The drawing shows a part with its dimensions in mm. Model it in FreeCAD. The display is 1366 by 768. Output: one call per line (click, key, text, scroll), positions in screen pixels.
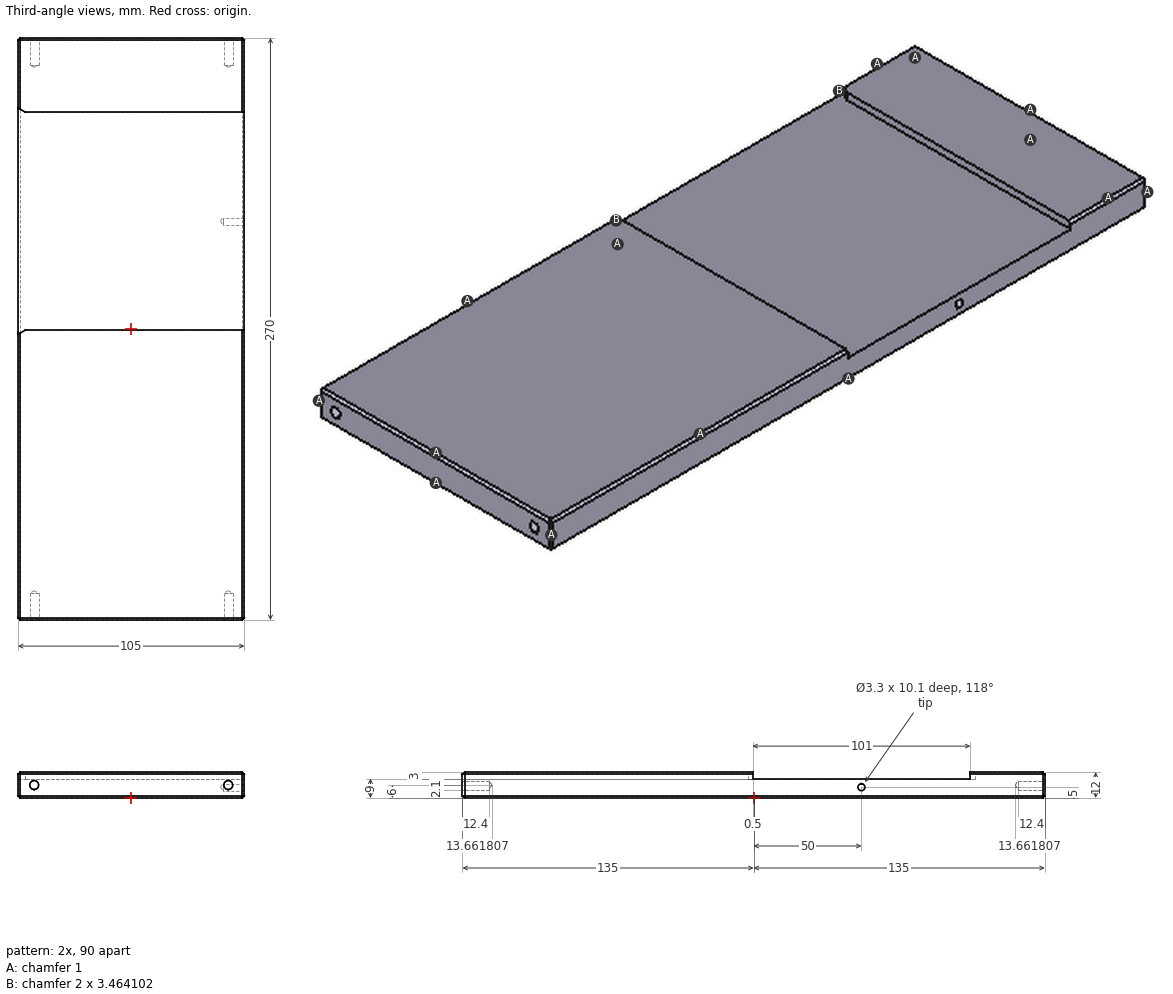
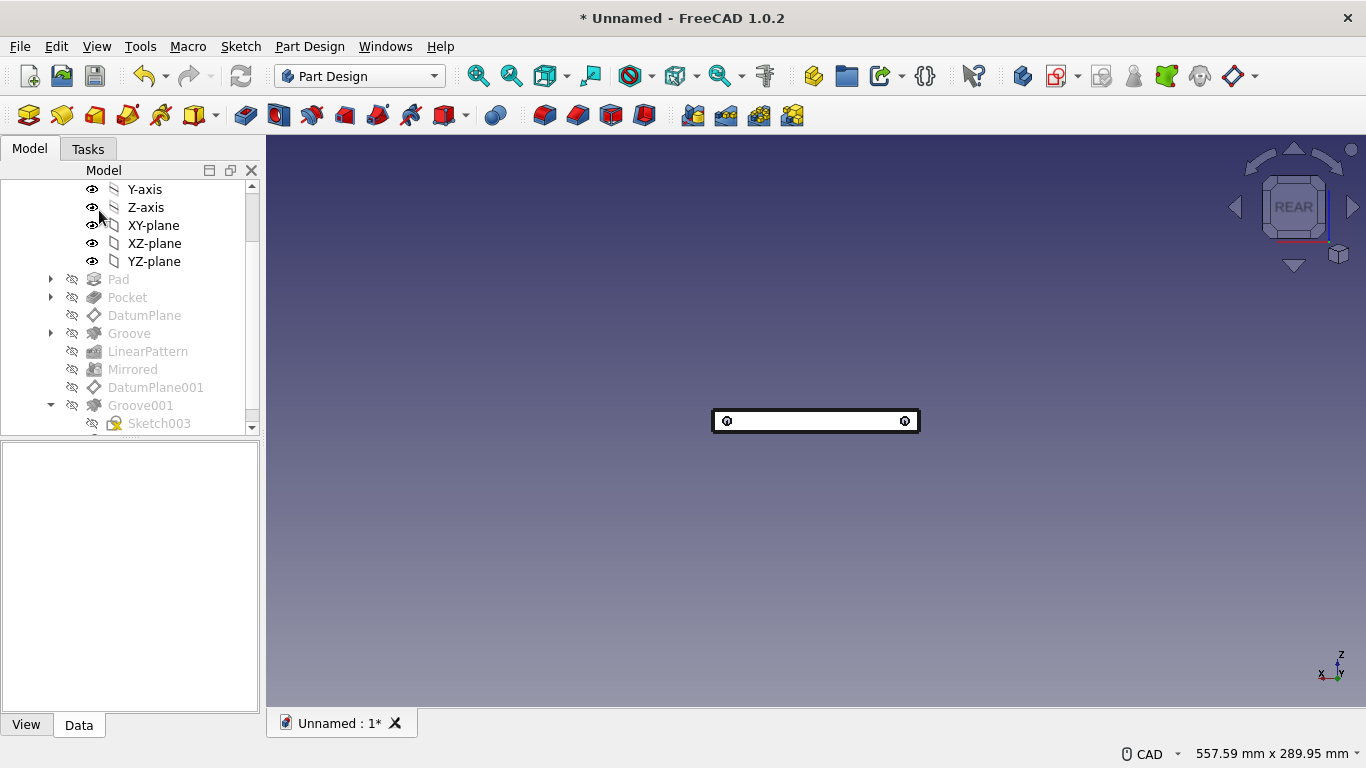
click(479, 76)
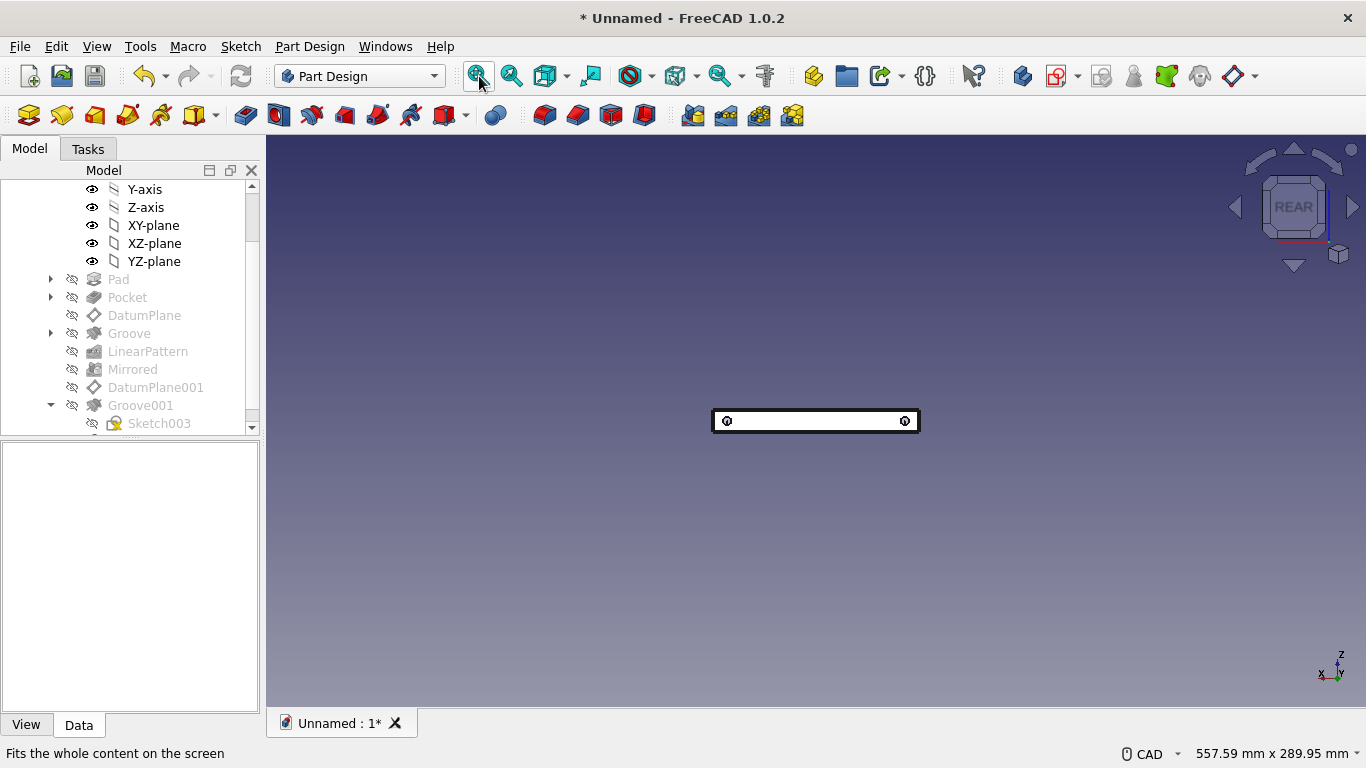
scroll(920, 412, up, 12)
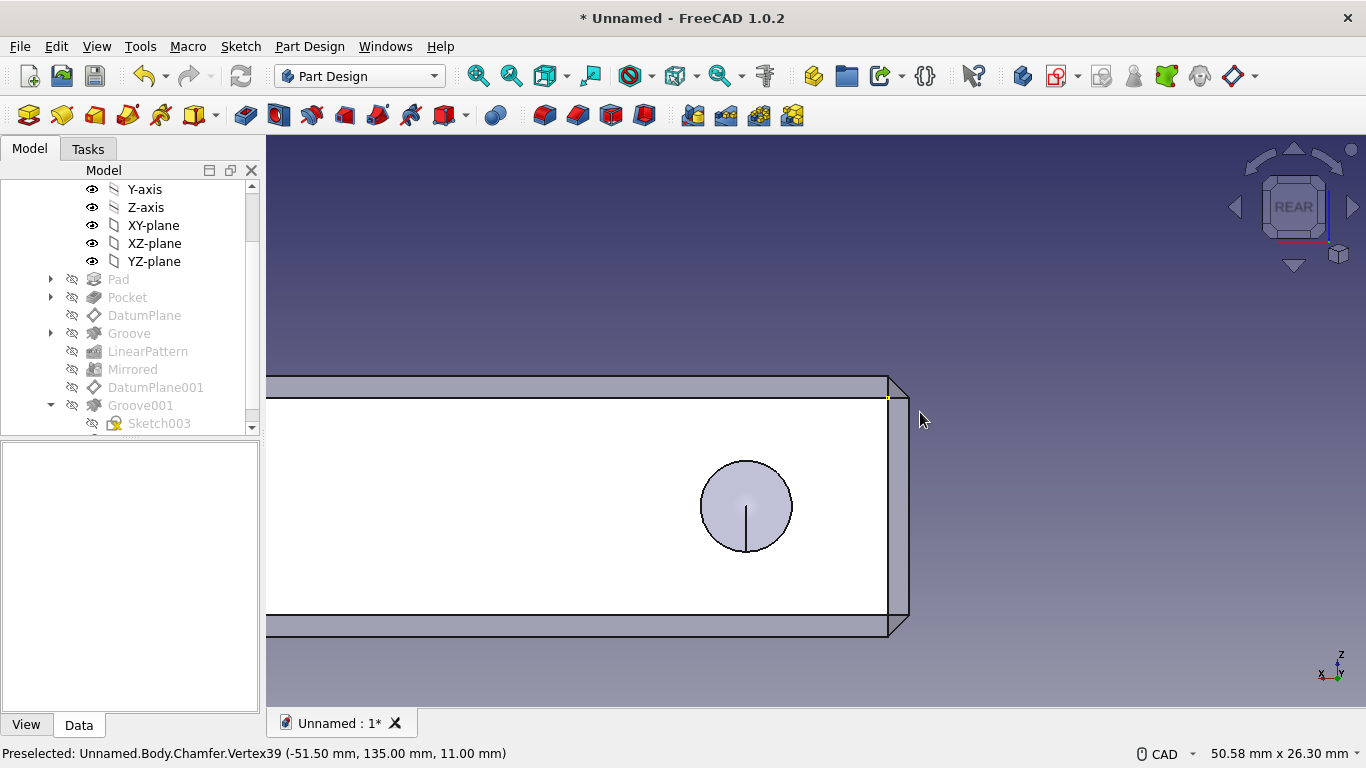
click(479, 76)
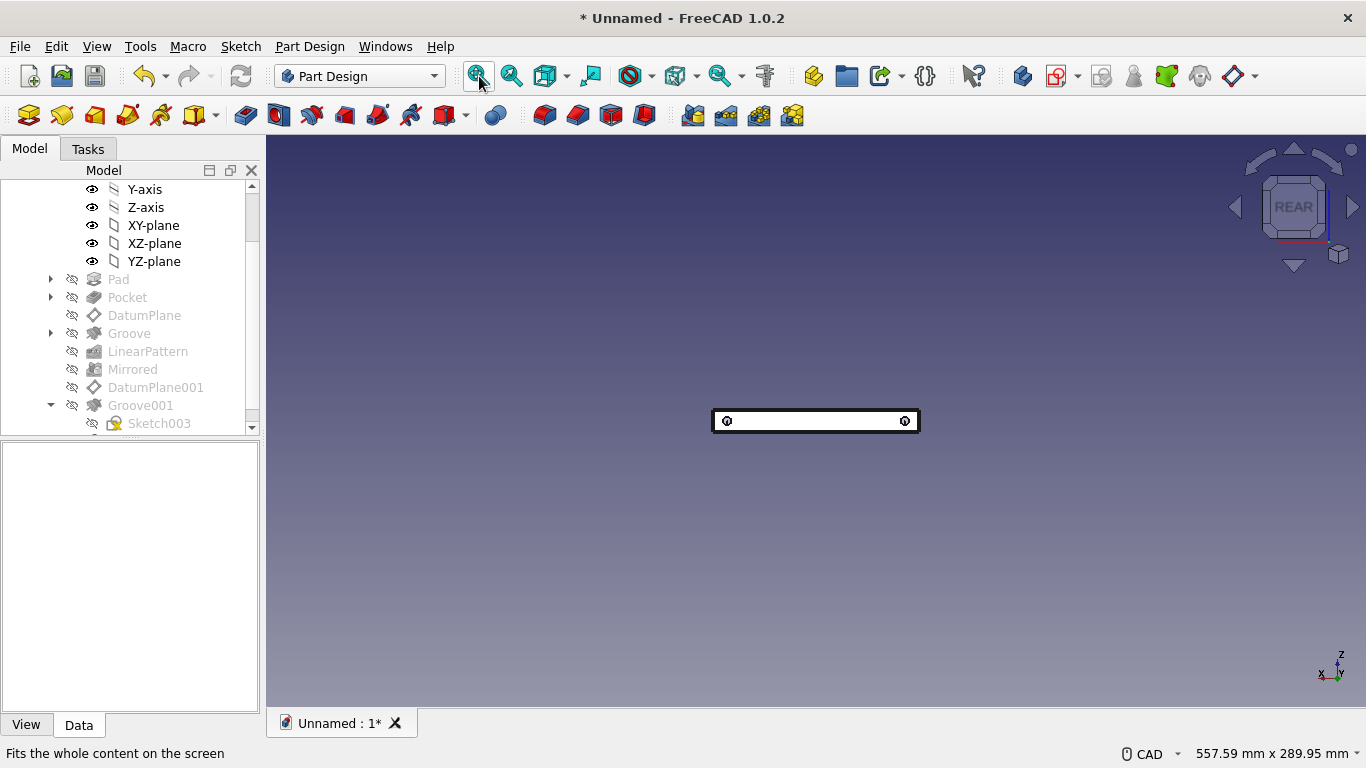
key(0)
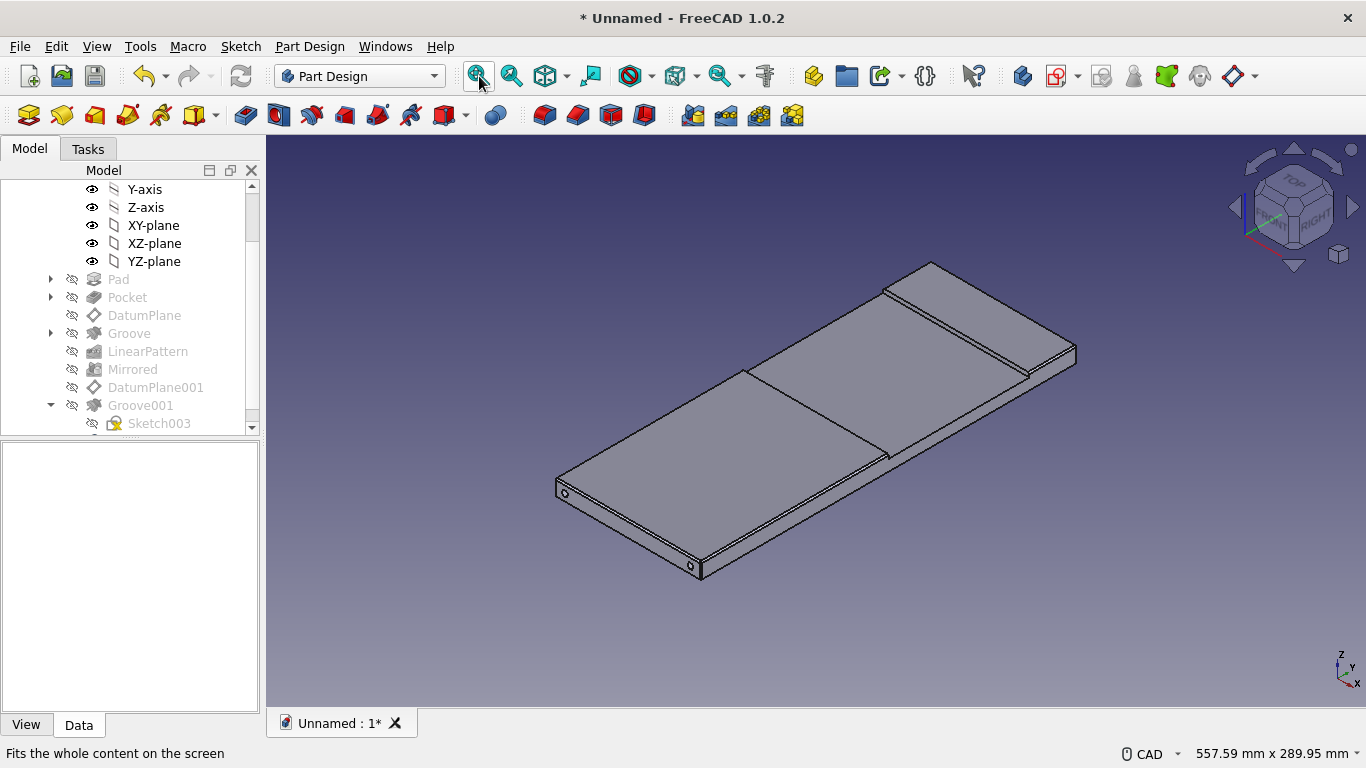
scroll(742, 372, up, 12)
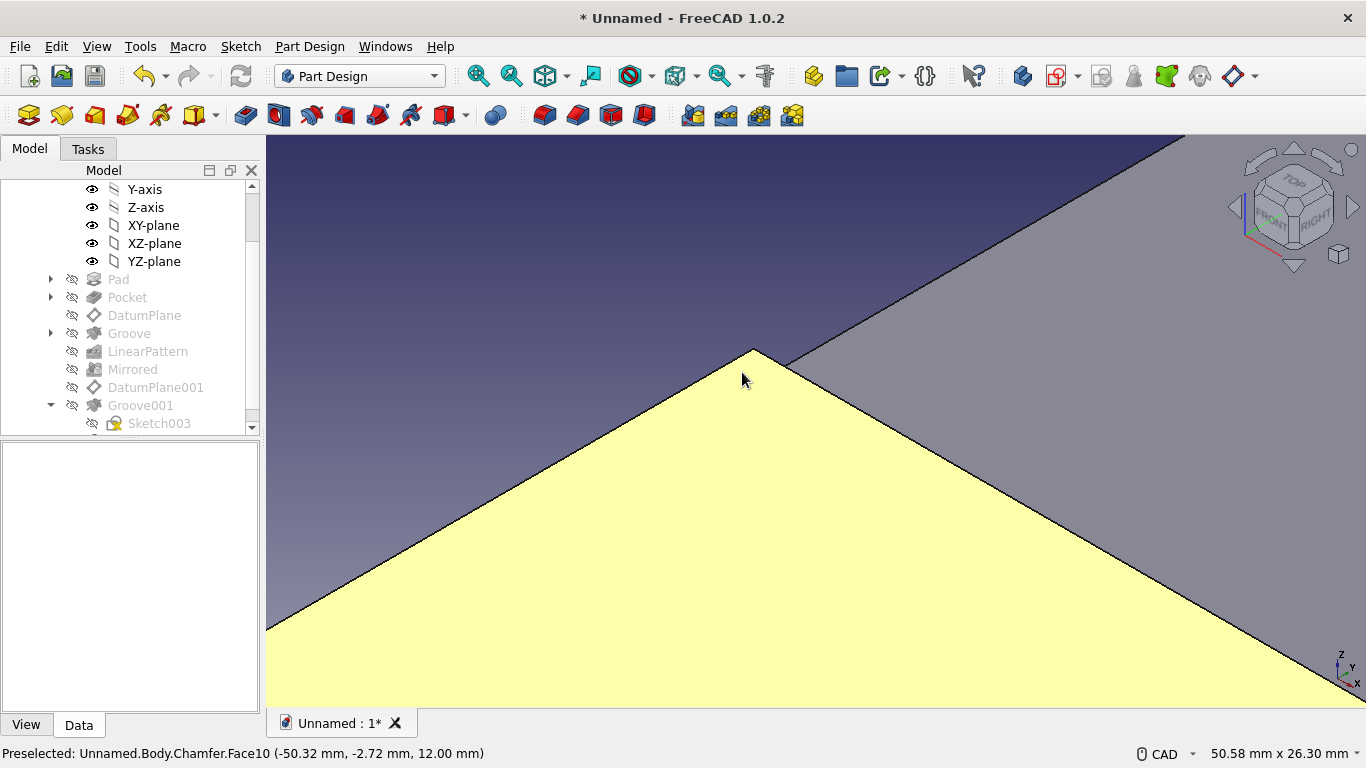
click(479, 76)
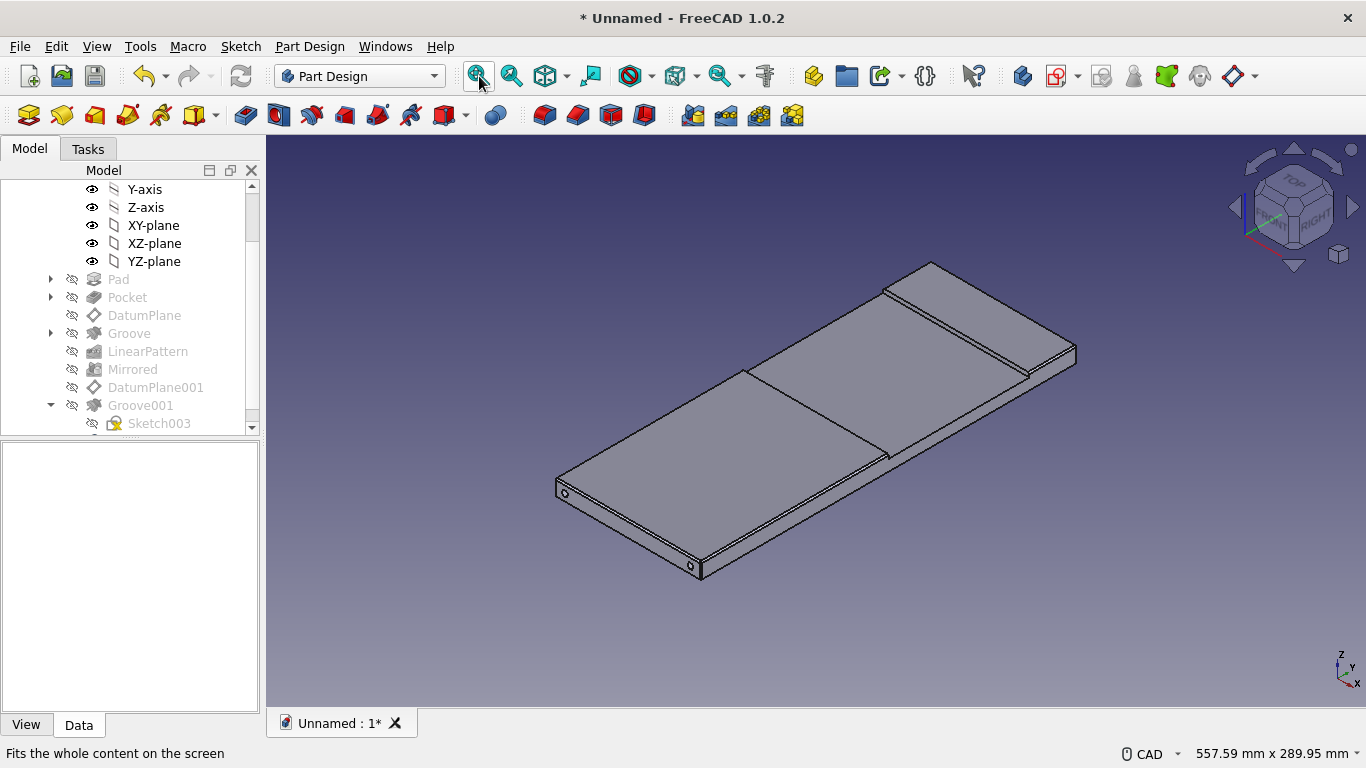
key(2)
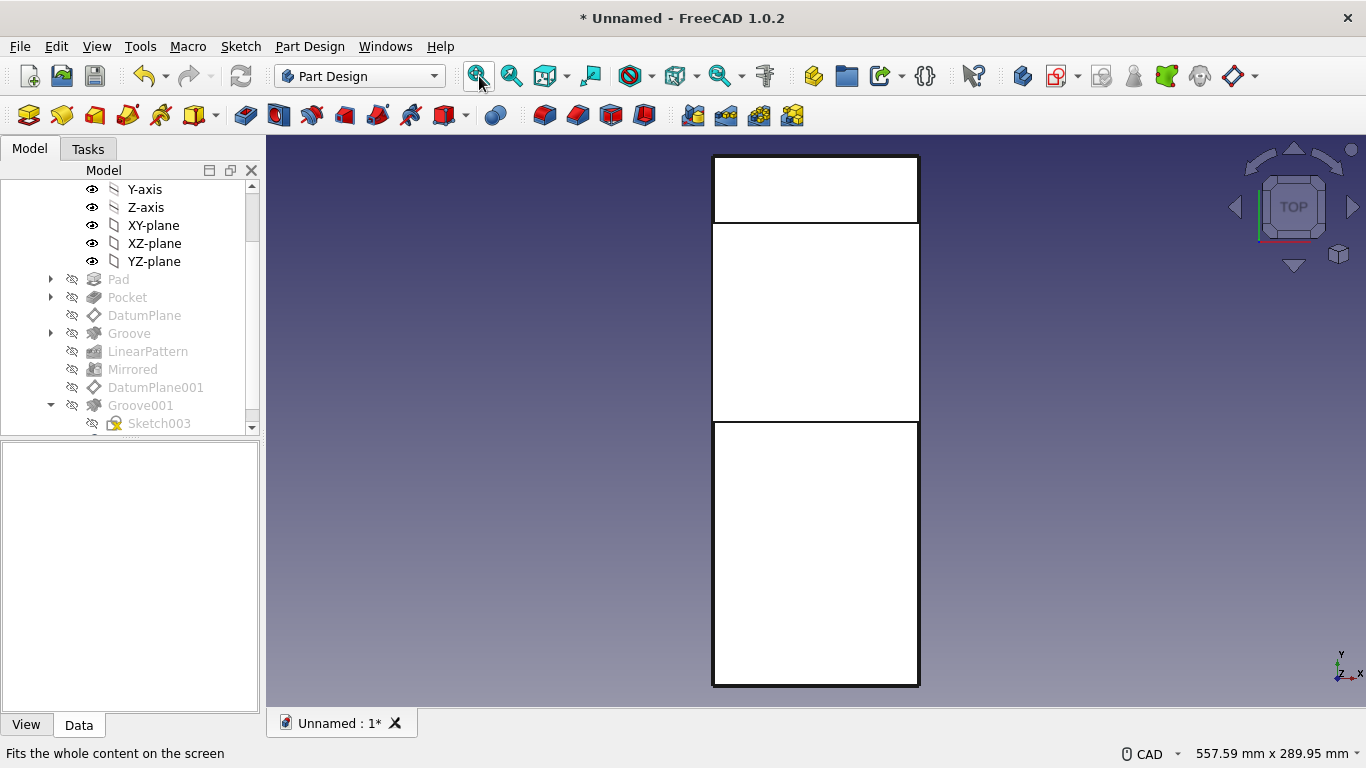
scroll(712, 421, up, 12)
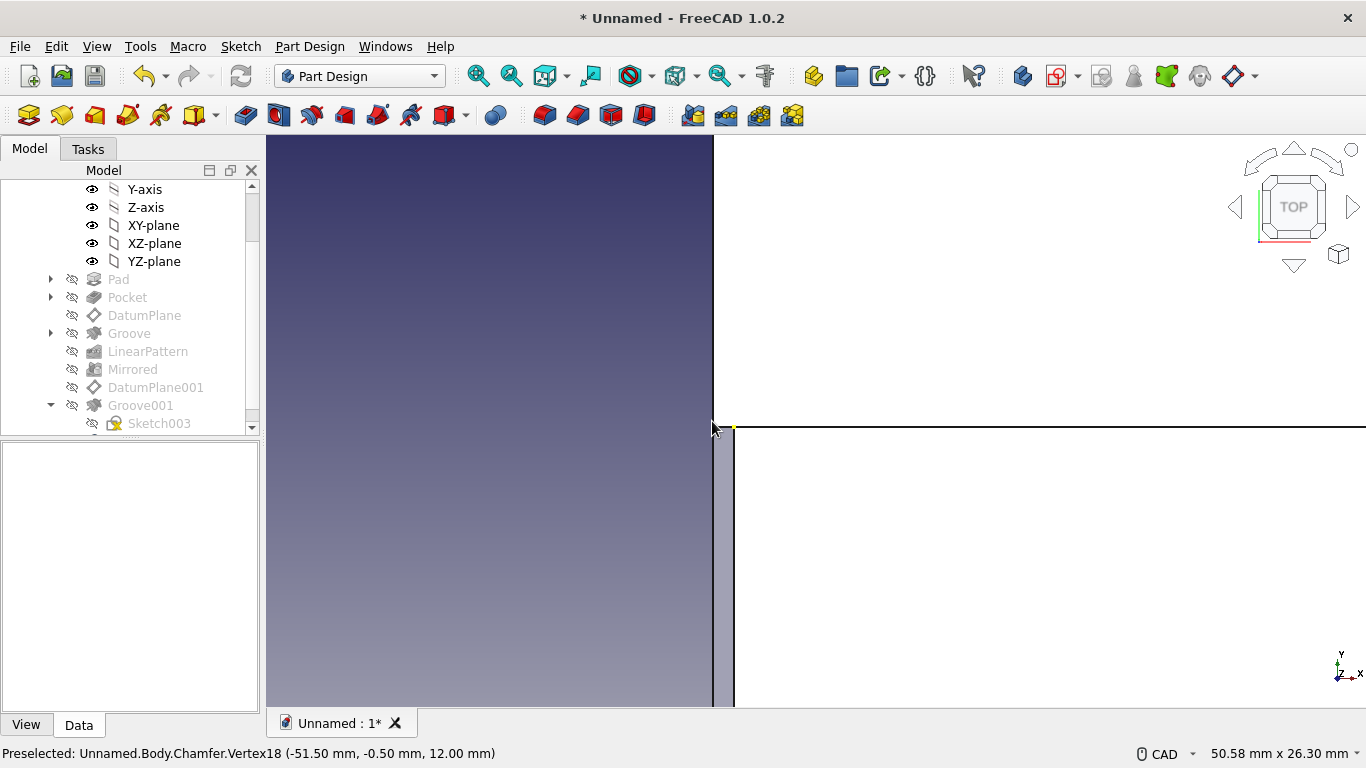
click(479, 76)